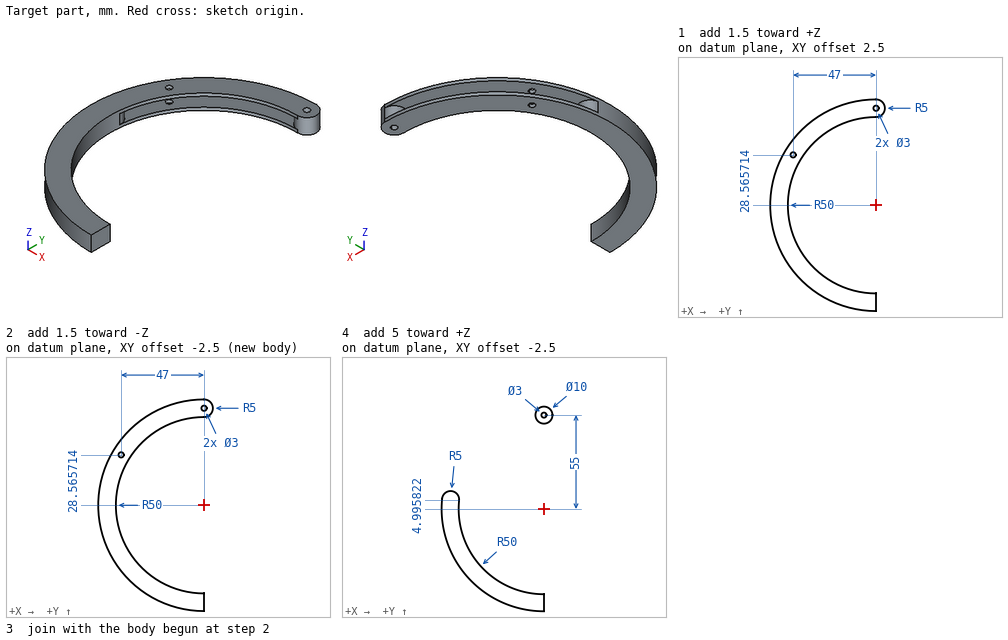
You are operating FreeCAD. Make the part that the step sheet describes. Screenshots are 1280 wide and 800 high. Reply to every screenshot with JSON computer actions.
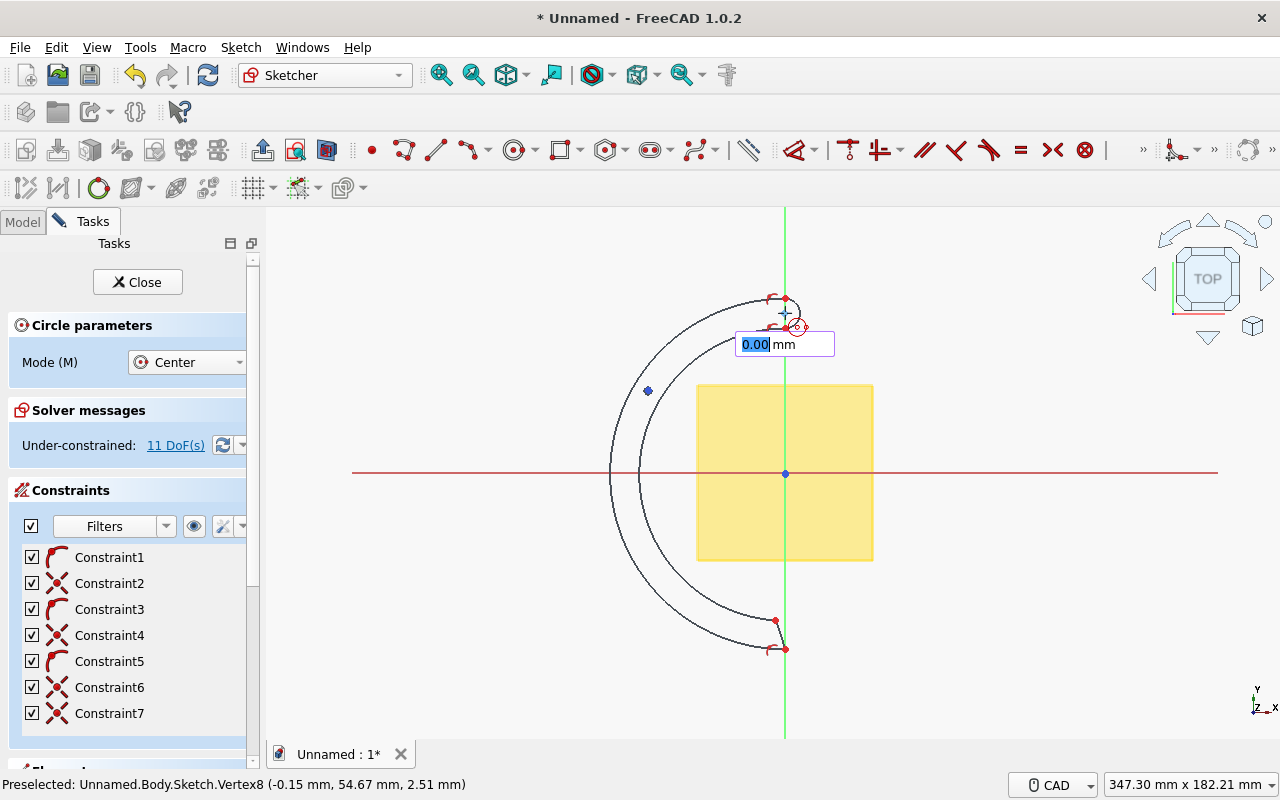
{"action": "scroll", "coordinate": [789, 311], "scroll_direction": "up", "scroll_amount": 7}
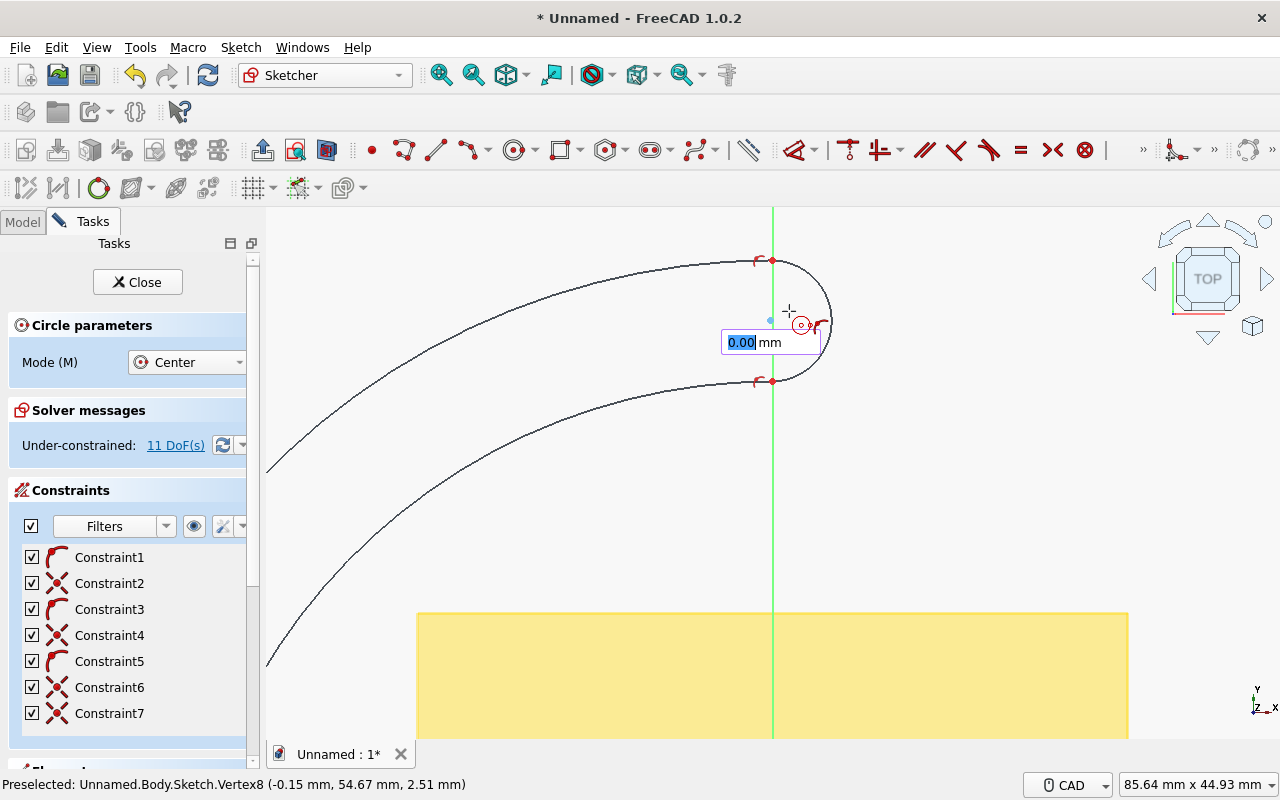
{"action": "left_click", "coordinate": [789, 311]}
{"action": "key", "text": "Escape"}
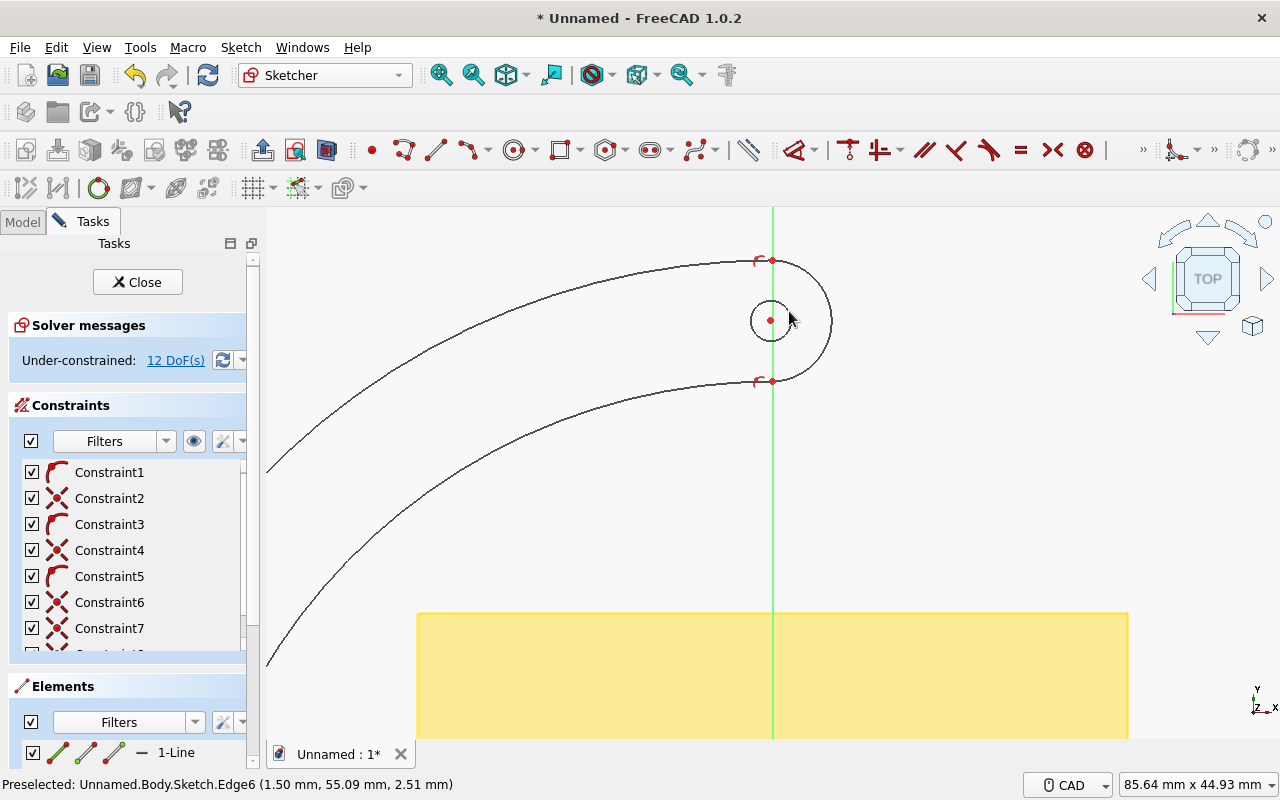
{"action": "scroll", "coordinate": [789, 311], "scroll_direction": "down", "scroll_amount": 7}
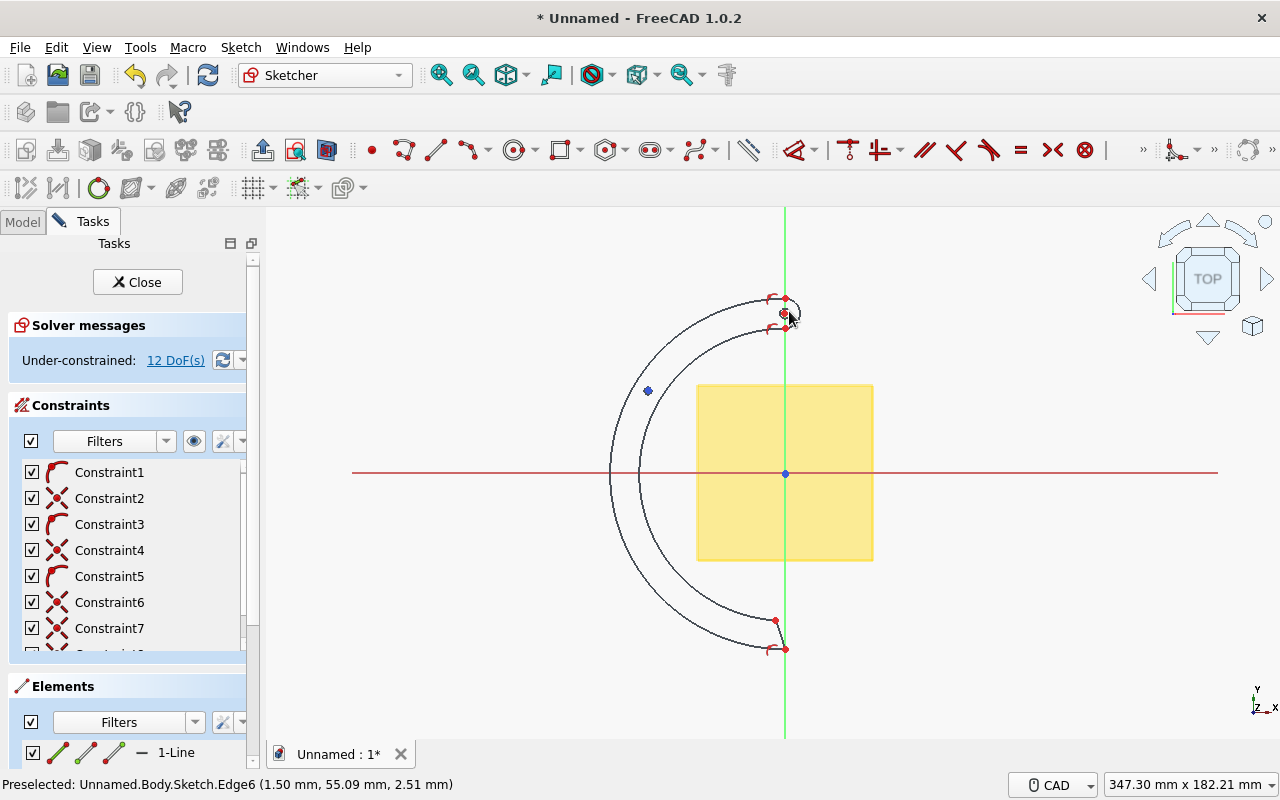
{"action": "left_click", "coordinate": [669, 386]}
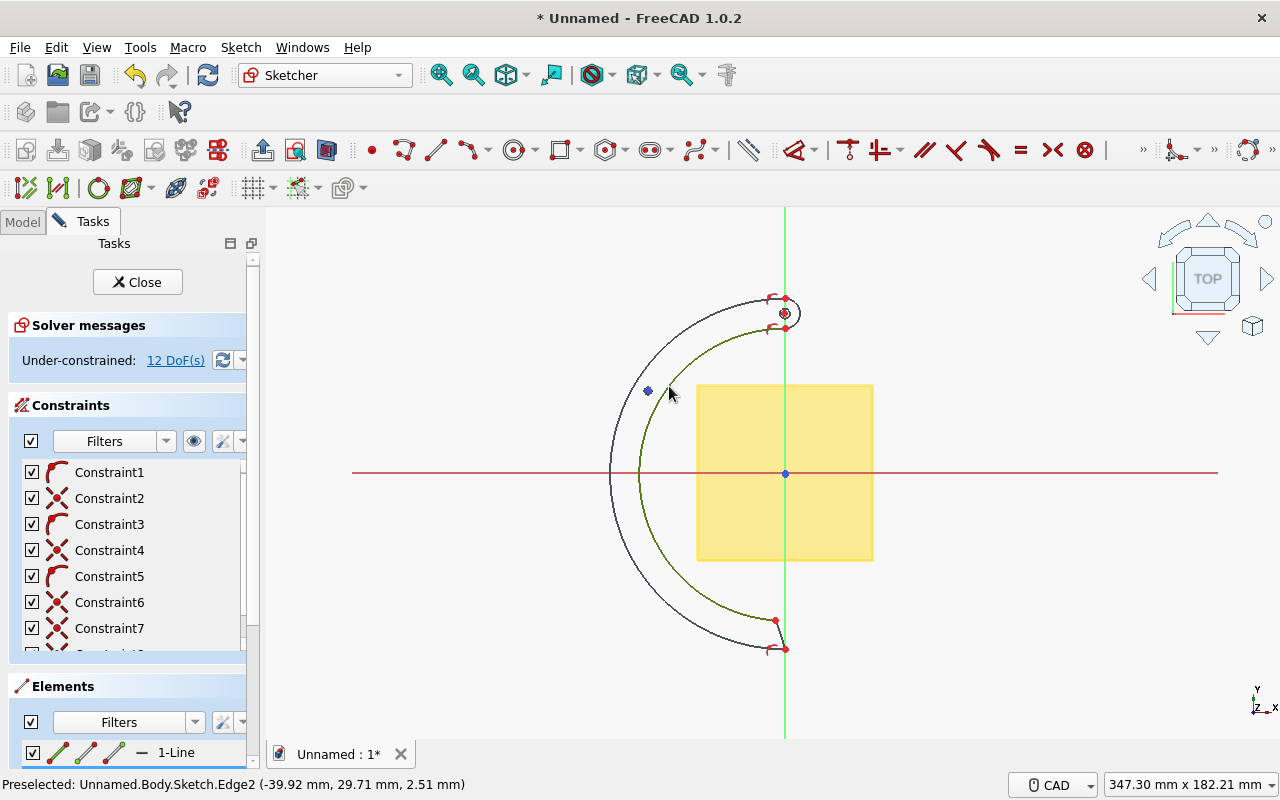
{"action": "scroll", "coordinate": [797, 322], "scroll_direction": "up", "scroll_amount": 2}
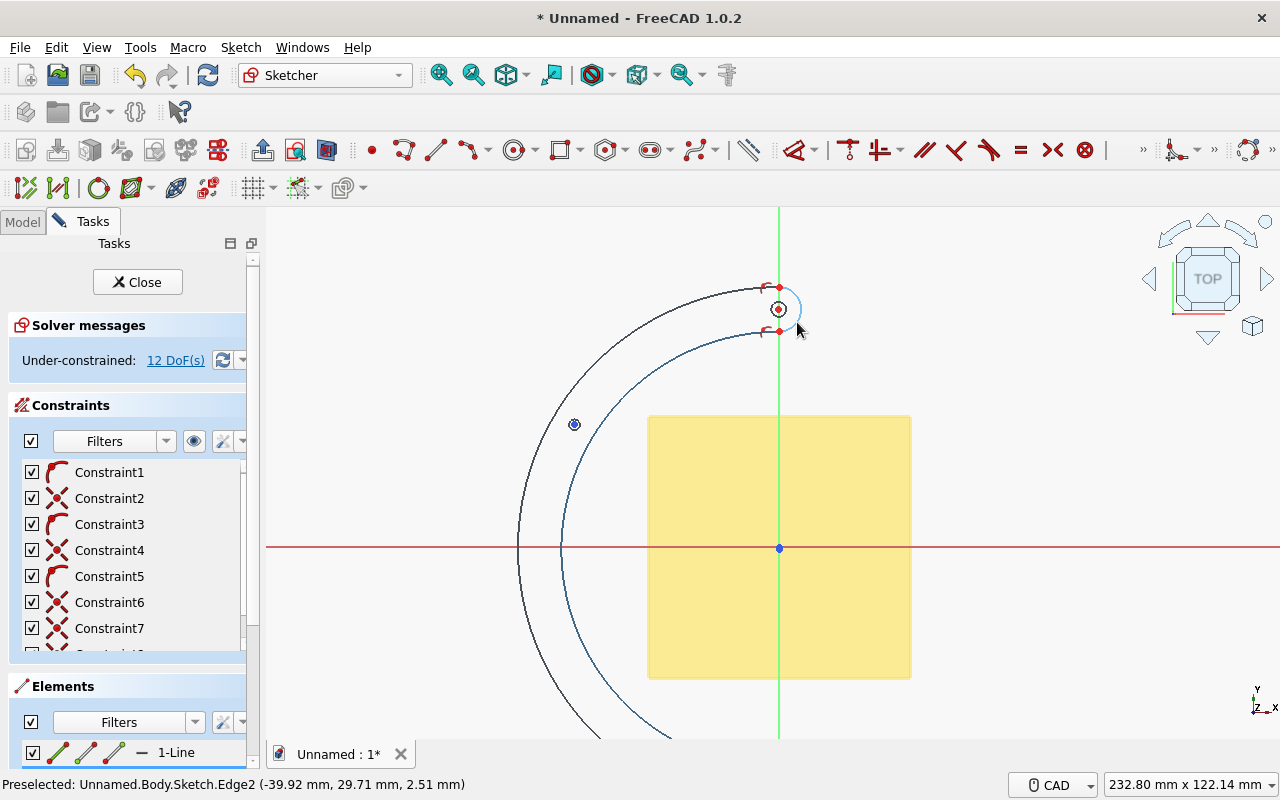
{"action": "left_click", "coordinate": [797, 322]}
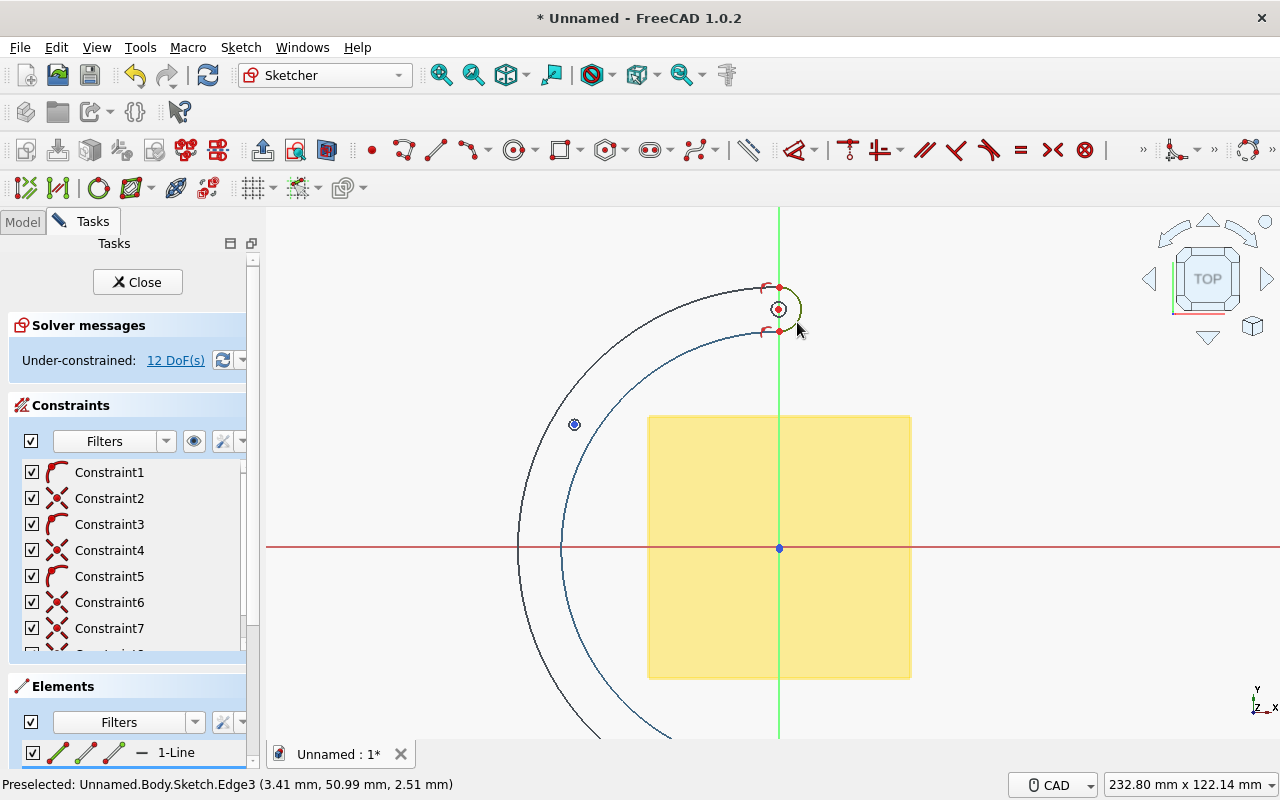
{"action": "left_click", "coordinate": [990, 150]}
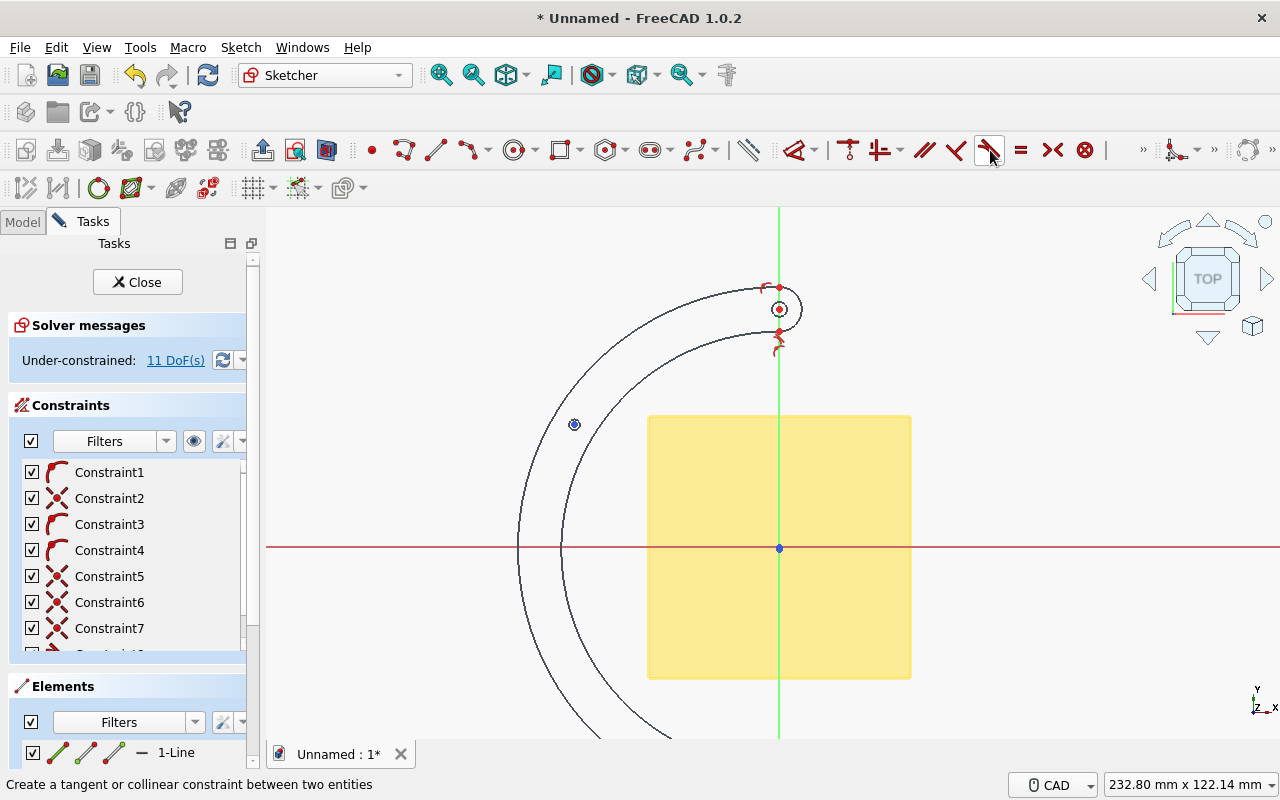
{"action": "scroll", "coordinate": [796, 322], "scroll_direction": "down", "scroll_amount": 2}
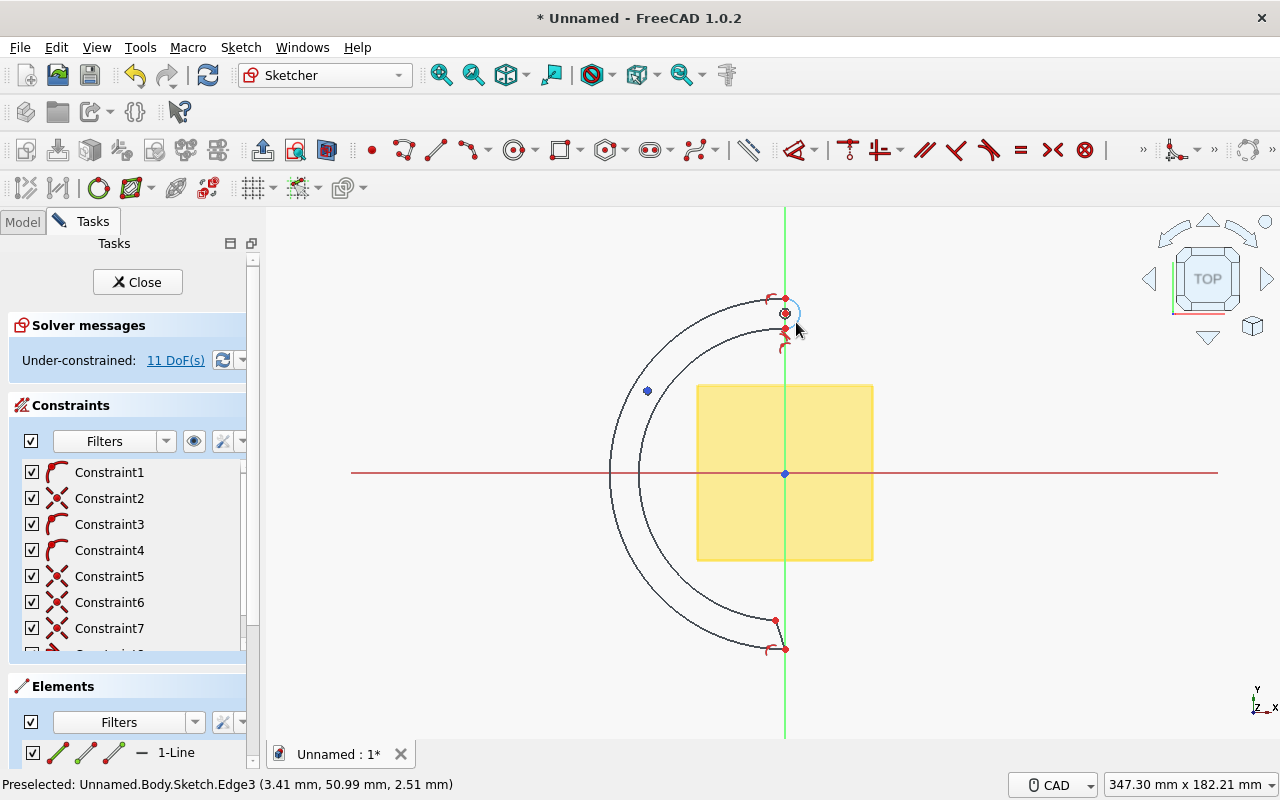
{"action": "scroll", "coordinate": [778, 629], "scroll_direction": "up", "scroll_amount": 4}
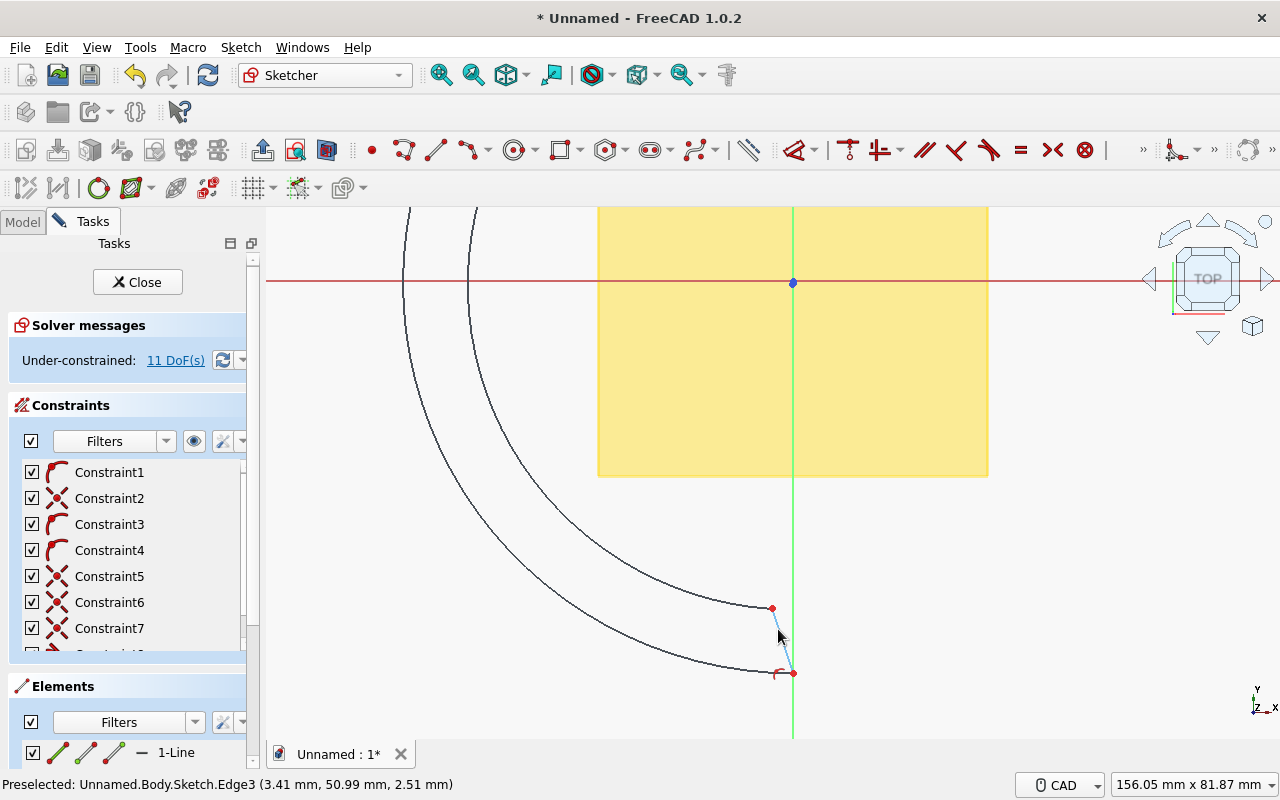
{"action": "left_click", "coordinate": [778, 628]}